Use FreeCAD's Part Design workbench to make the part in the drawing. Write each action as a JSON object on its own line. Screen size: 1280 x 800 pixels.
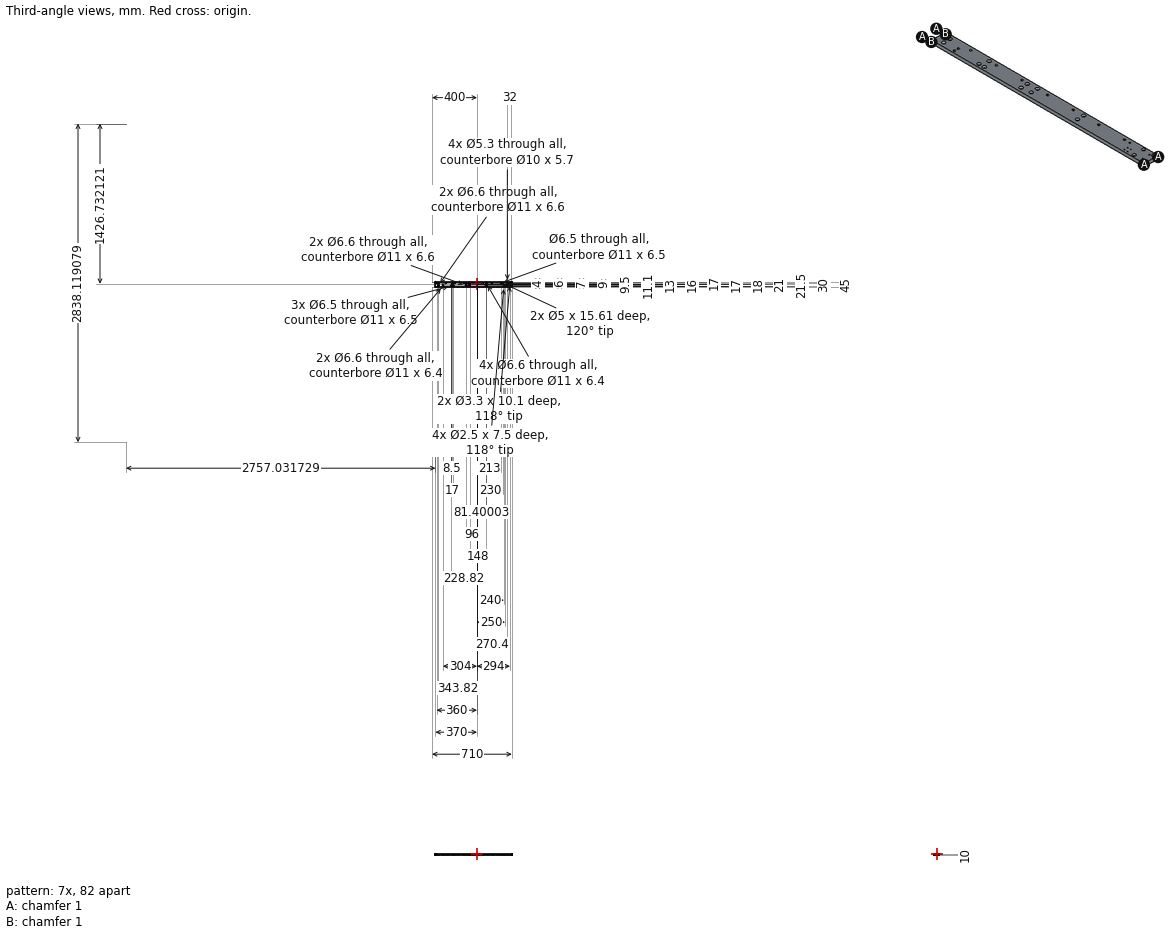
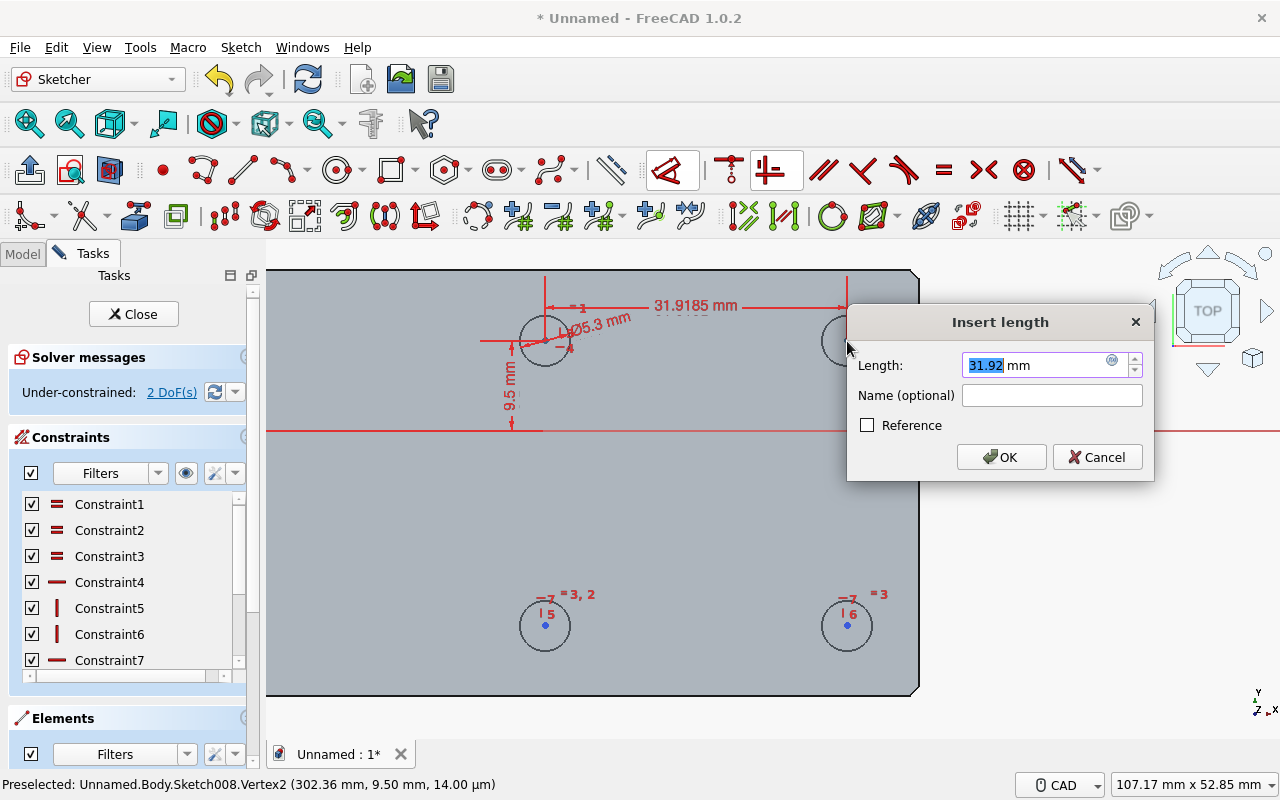
{"action": "type", "text": "32"}
{"action": "key", "text": "Return"}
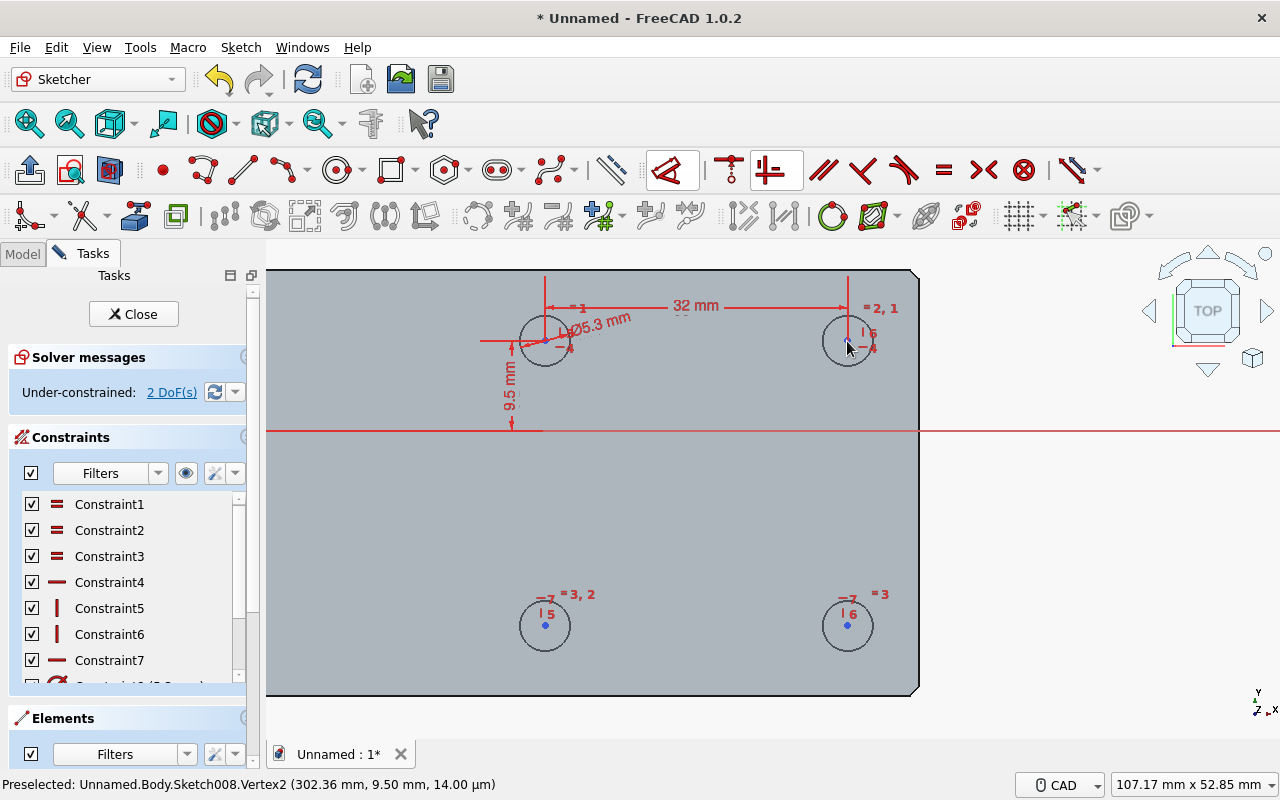
{"action": "left_click", "coordinate": [545, 341]}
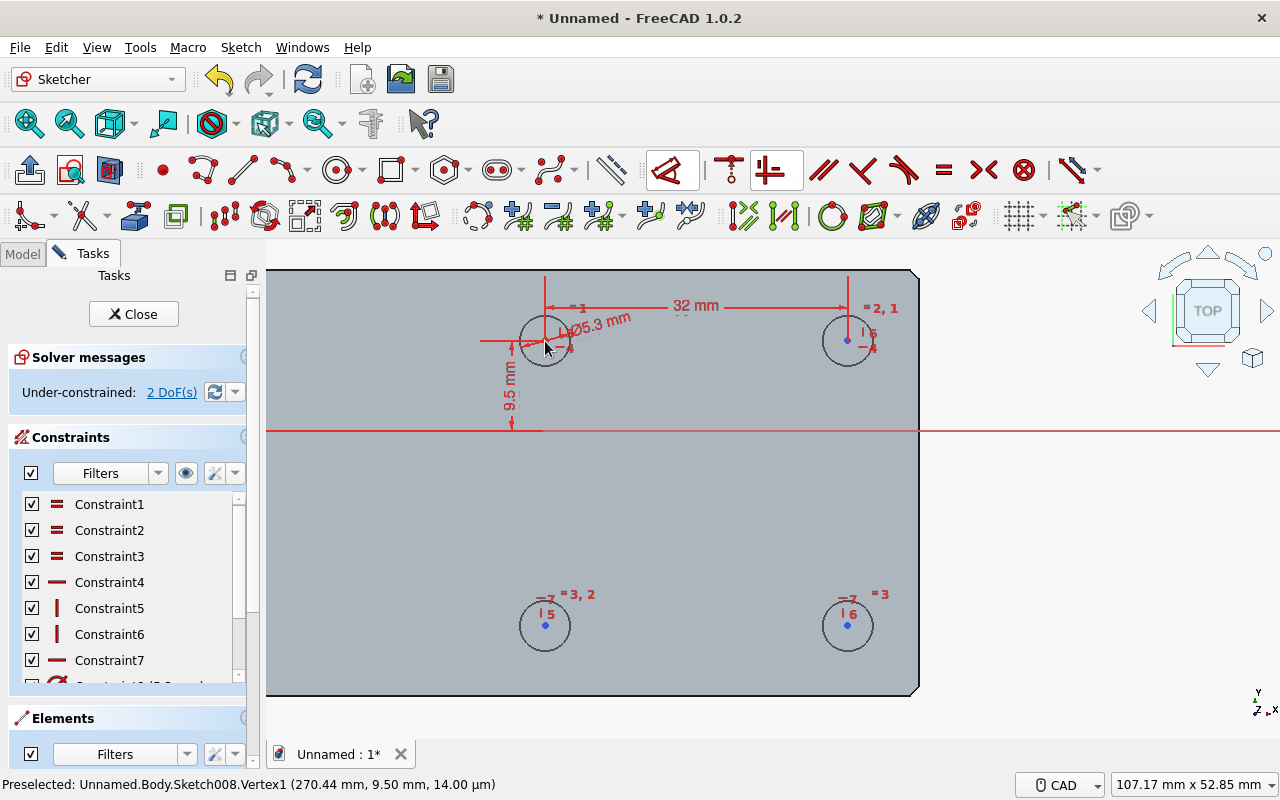
{"action": "left_click", "coordinate": [545, 626]}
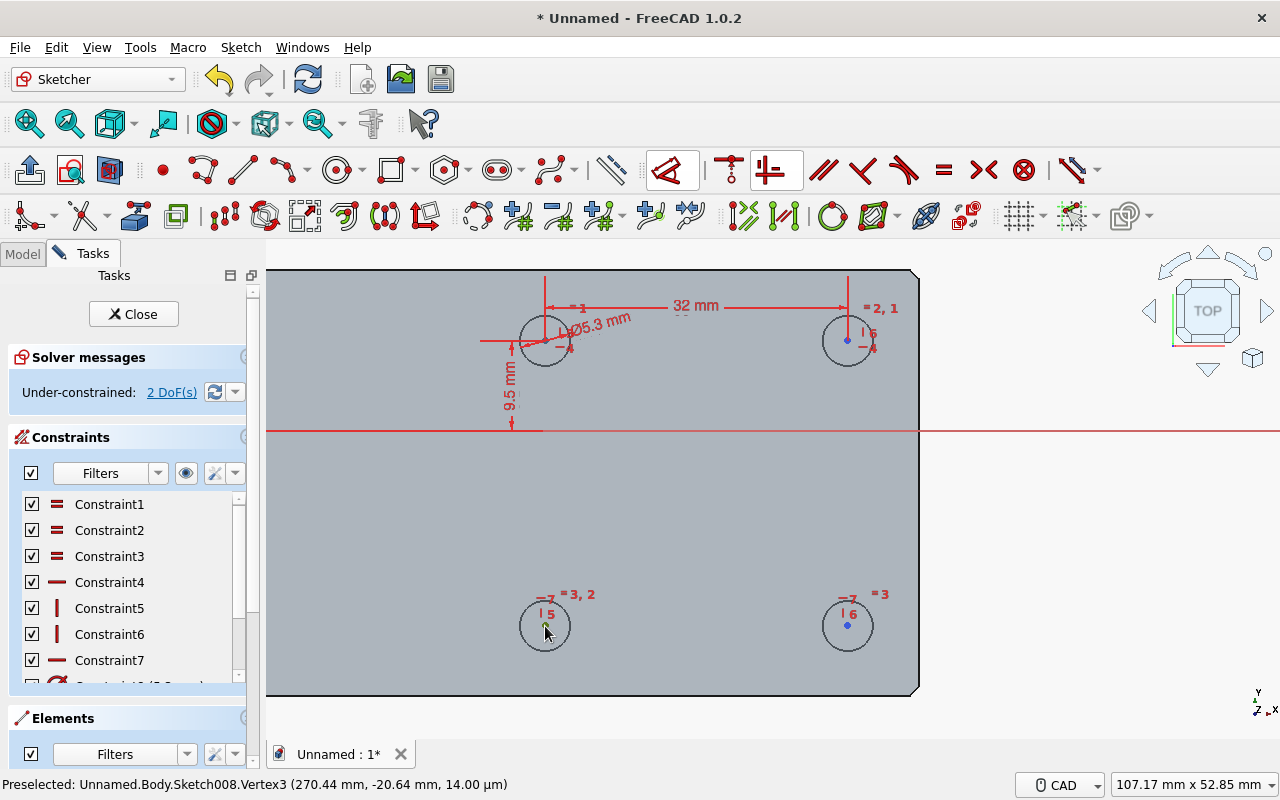
{"action": "key", "text": "i"}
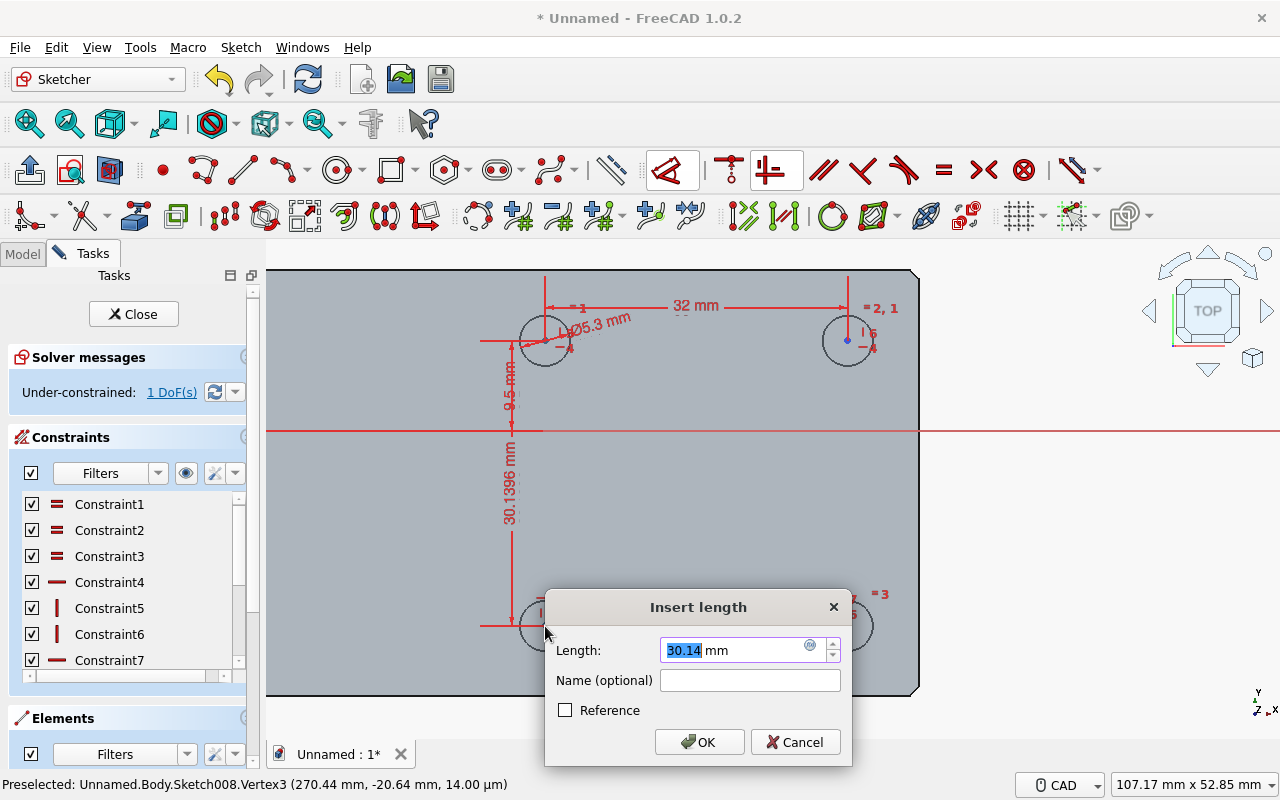
{"action": "type", "text": "30"}
{"action": "key", "text": "Return"}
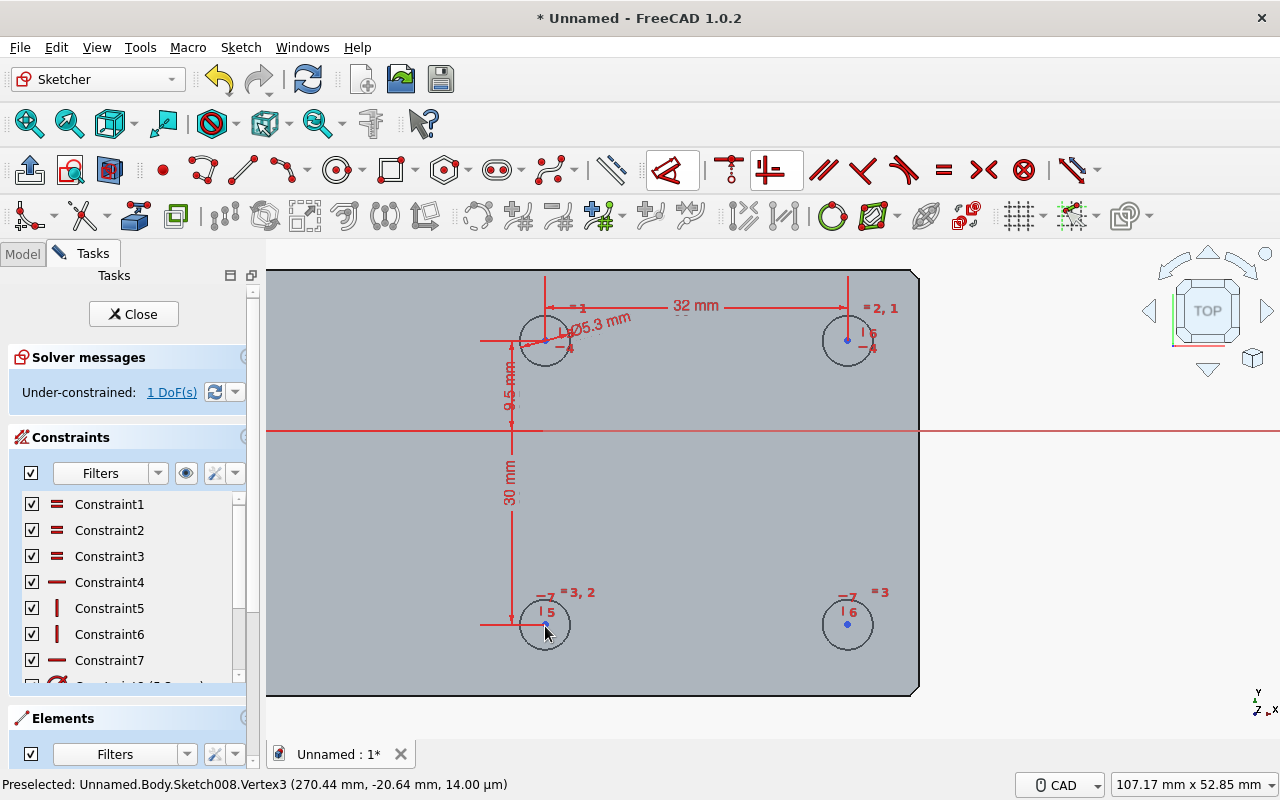
{"action": "left_click", "coordinate": [545, 341]}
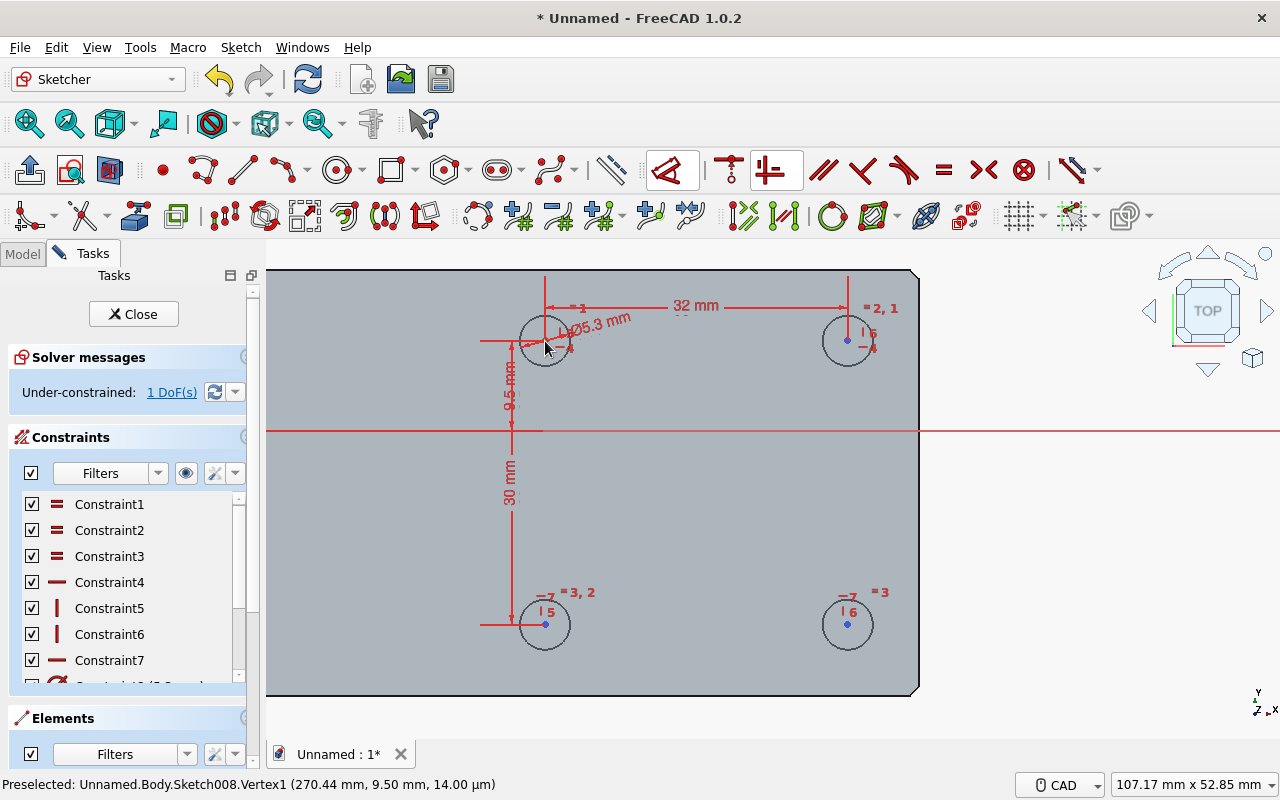
{"action": "left_click", "coordinate": [694, 170]}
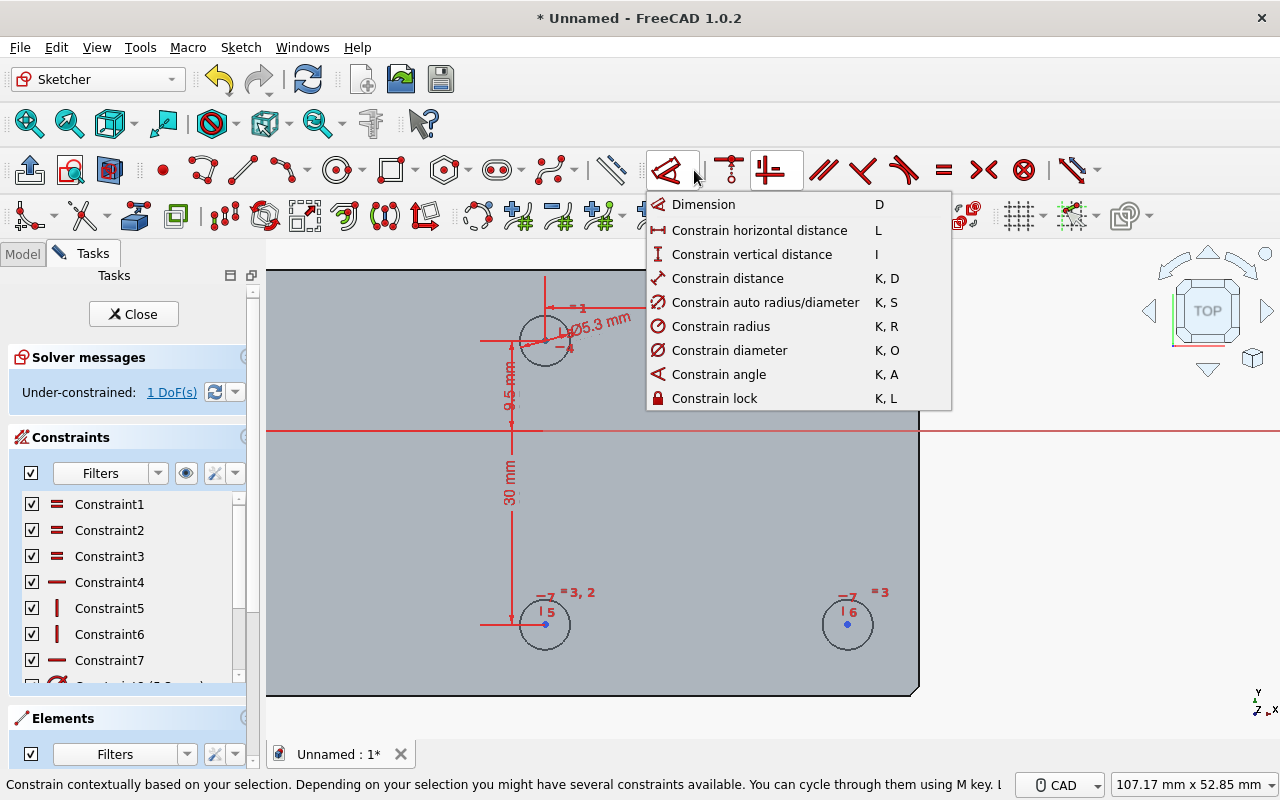
{"action": "left_click", "coordinate": [799, 230]}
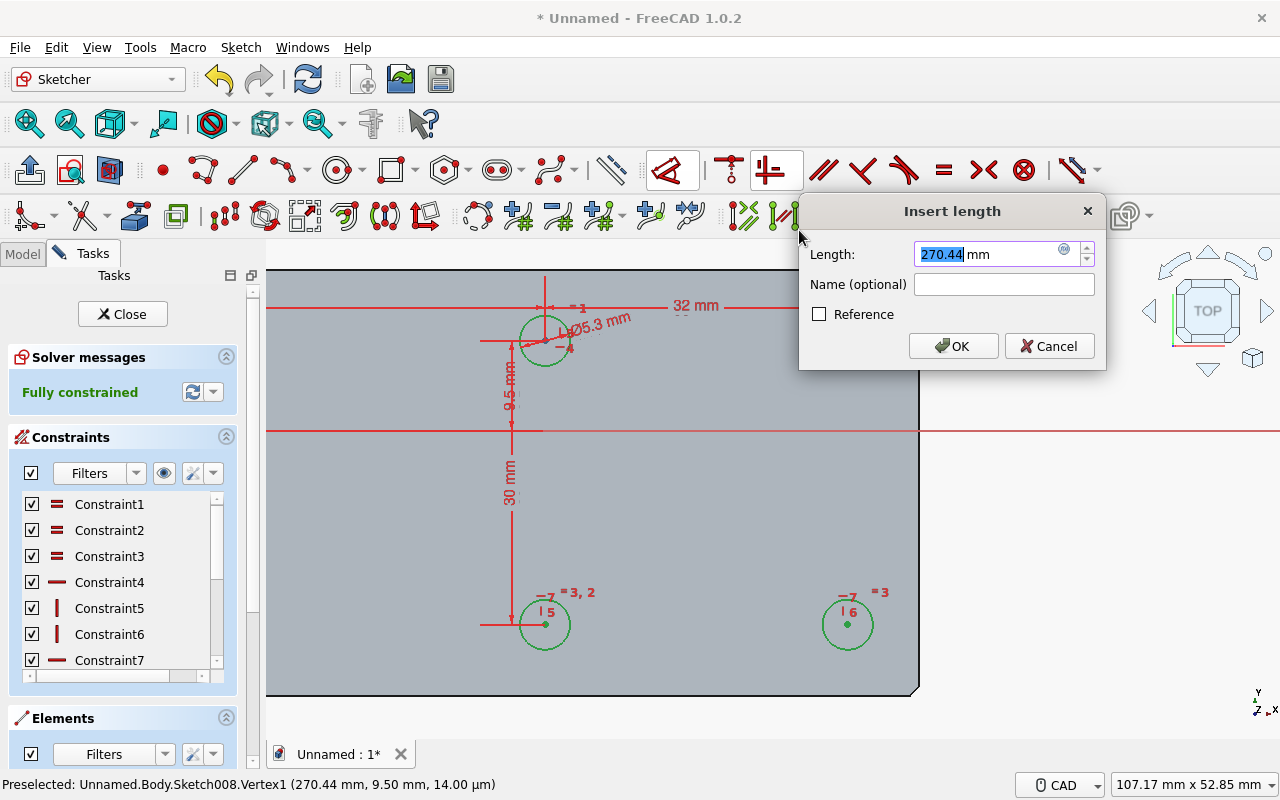
{"action": "type", "text": "270.4"}
{"action": "key", "text": "Return"}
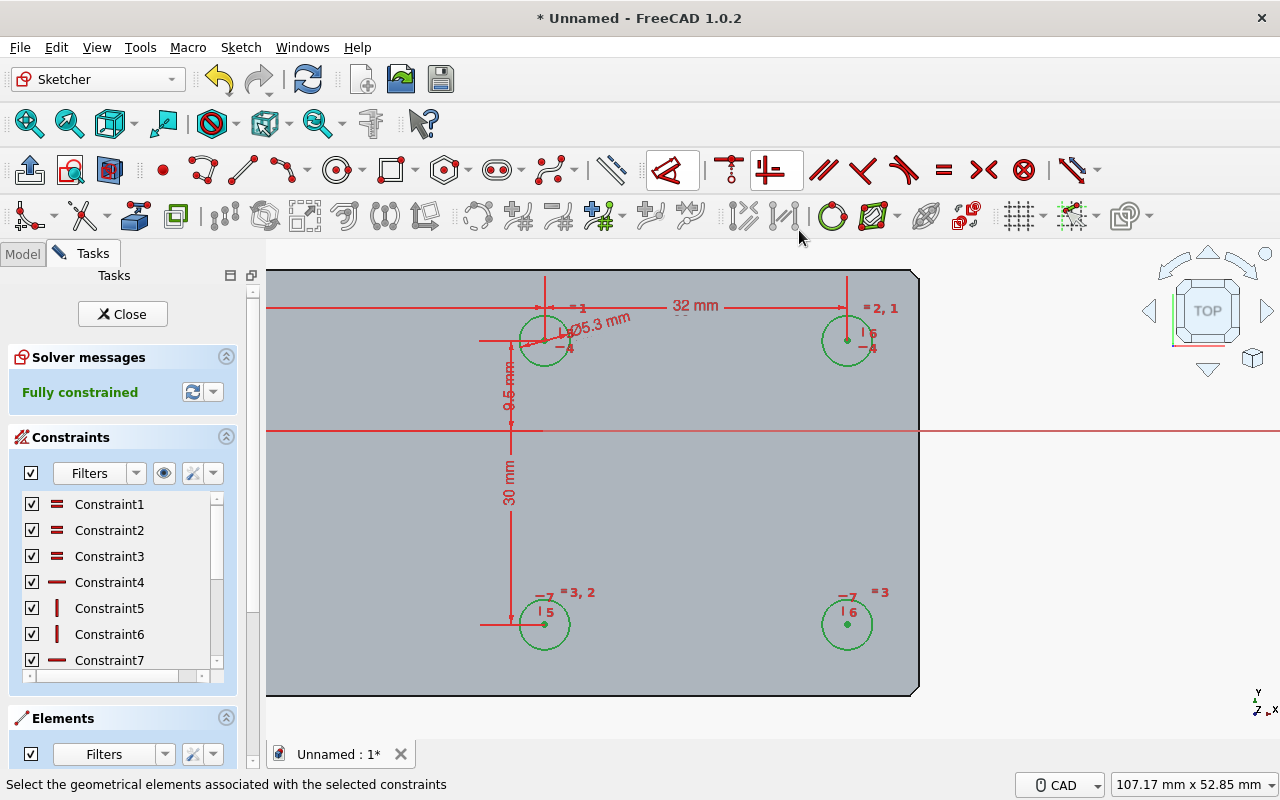
{"action": "left_click", "coordinate": [123, 314]}